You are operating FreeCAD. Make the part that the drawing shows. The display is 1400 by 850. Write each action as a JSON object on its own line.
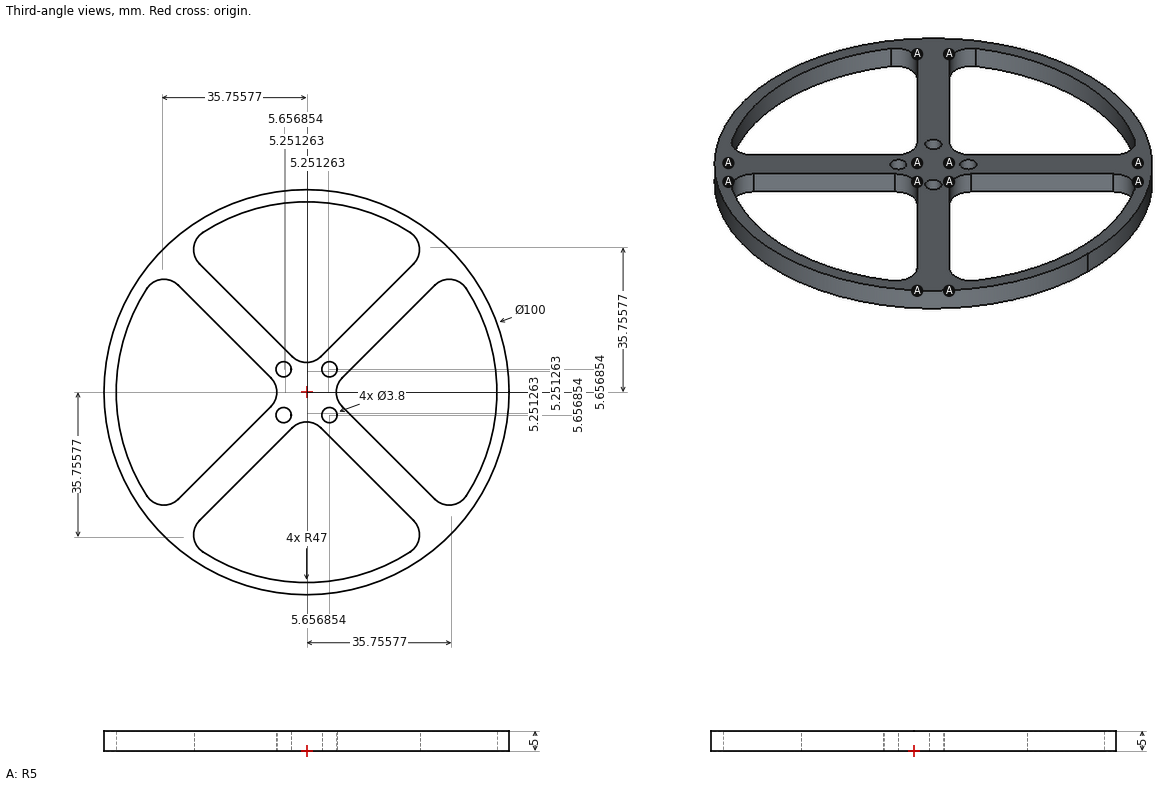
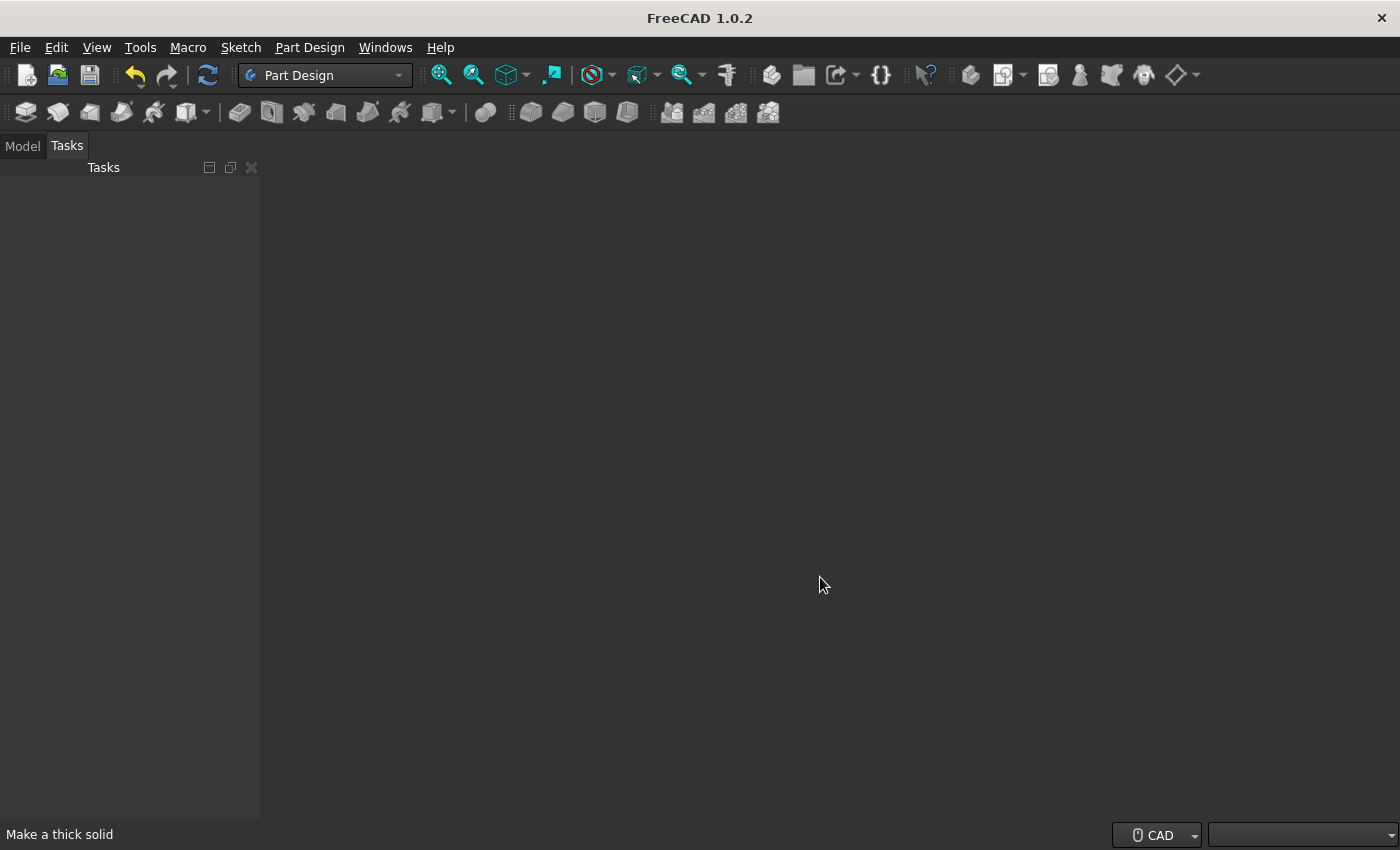
{"action": "left_click", "coordinate": [26, 76]}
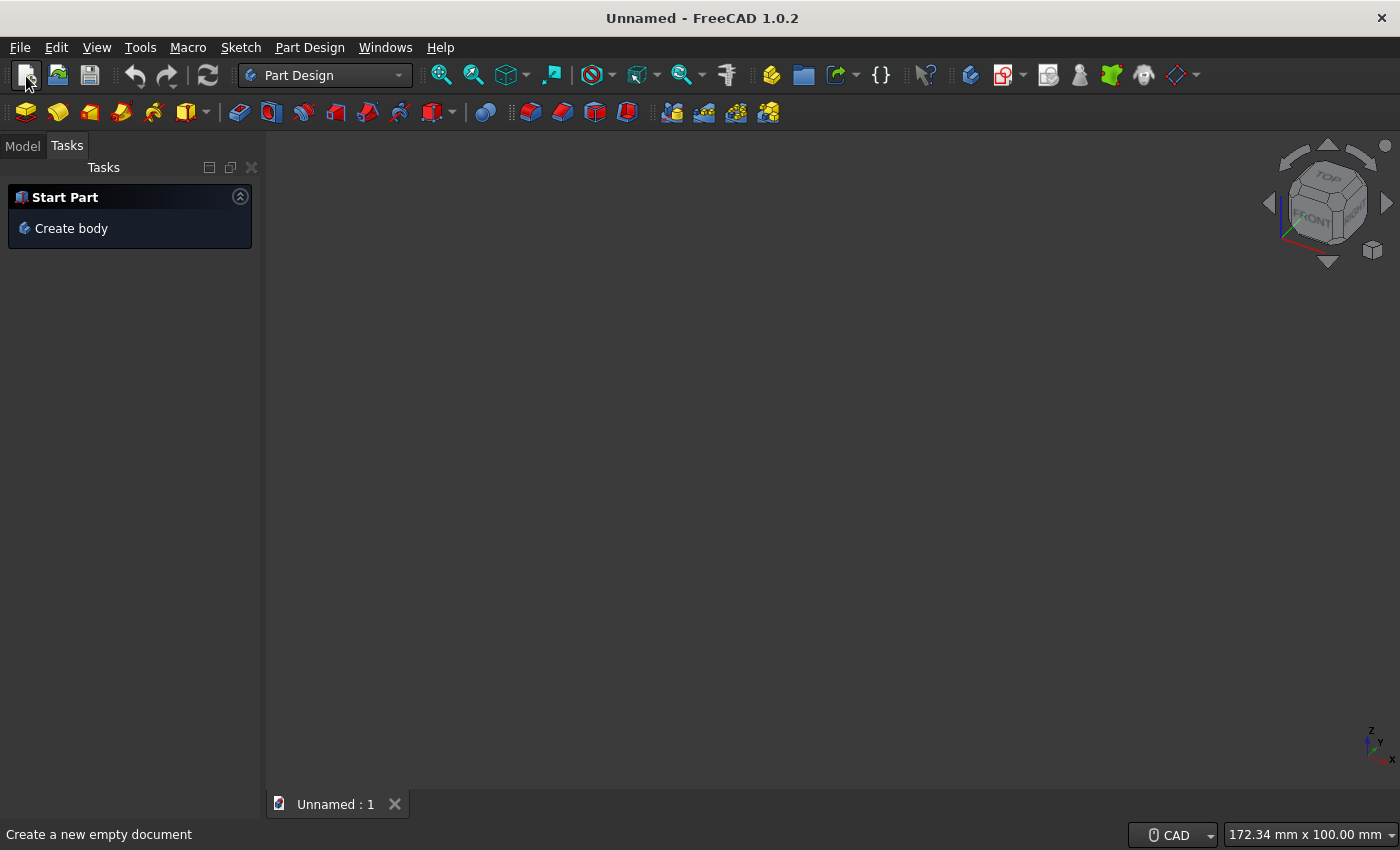
{"action": "left_click", "coordinate": [1004, 76]}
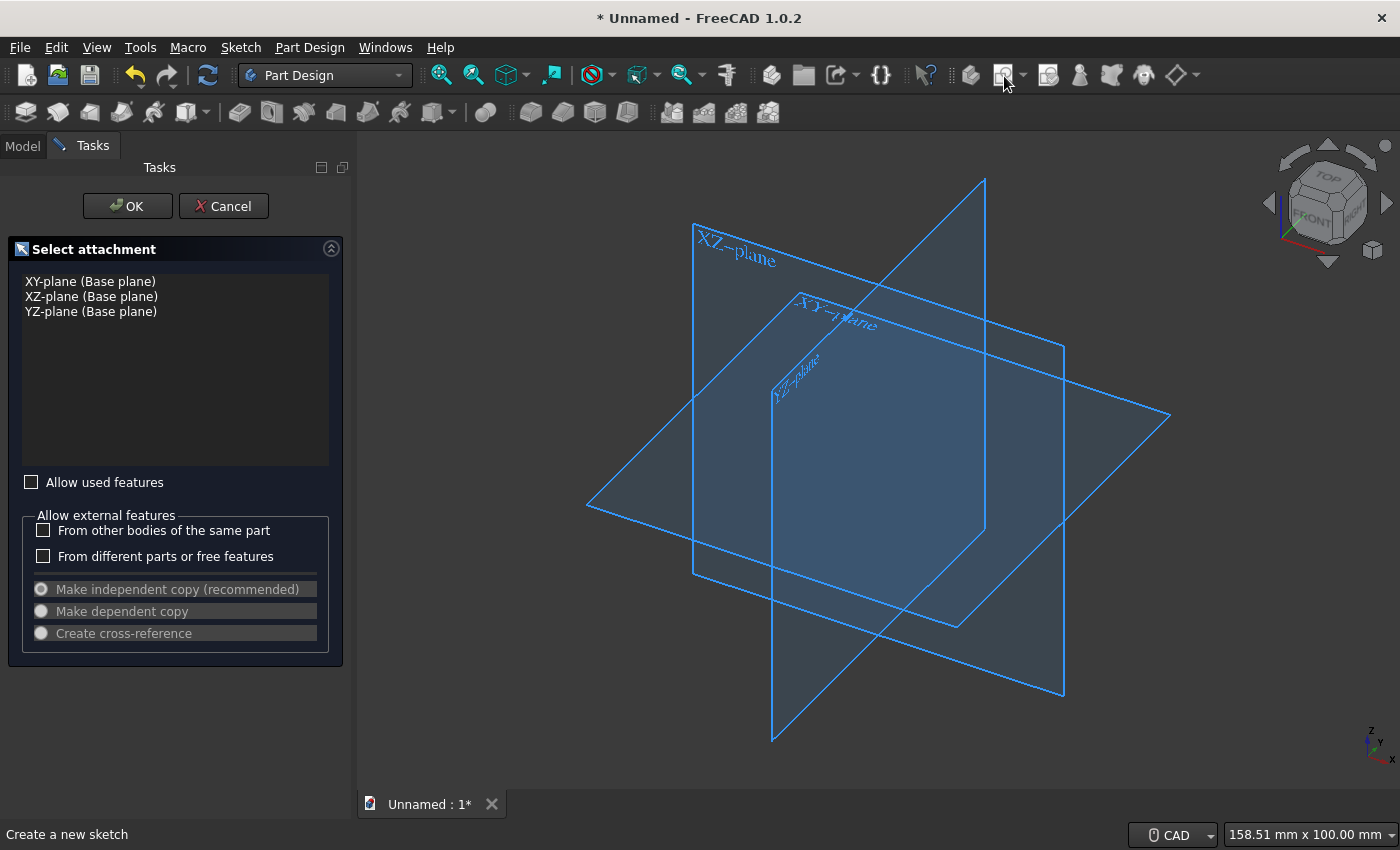
{"action": "left_click", "coordinate": [82, 282]}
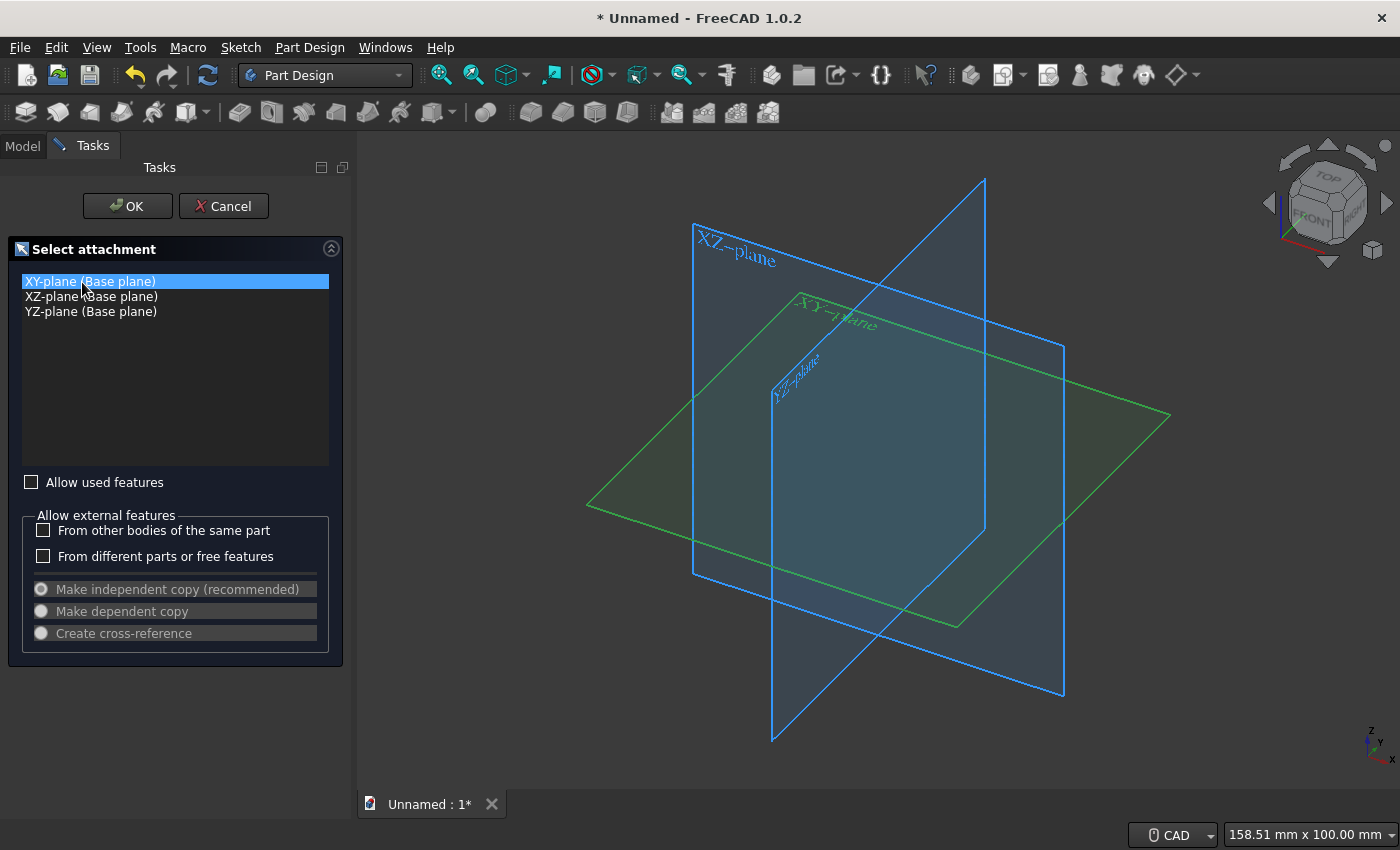
{"action": "left_click", "coordinate": [128, 206]}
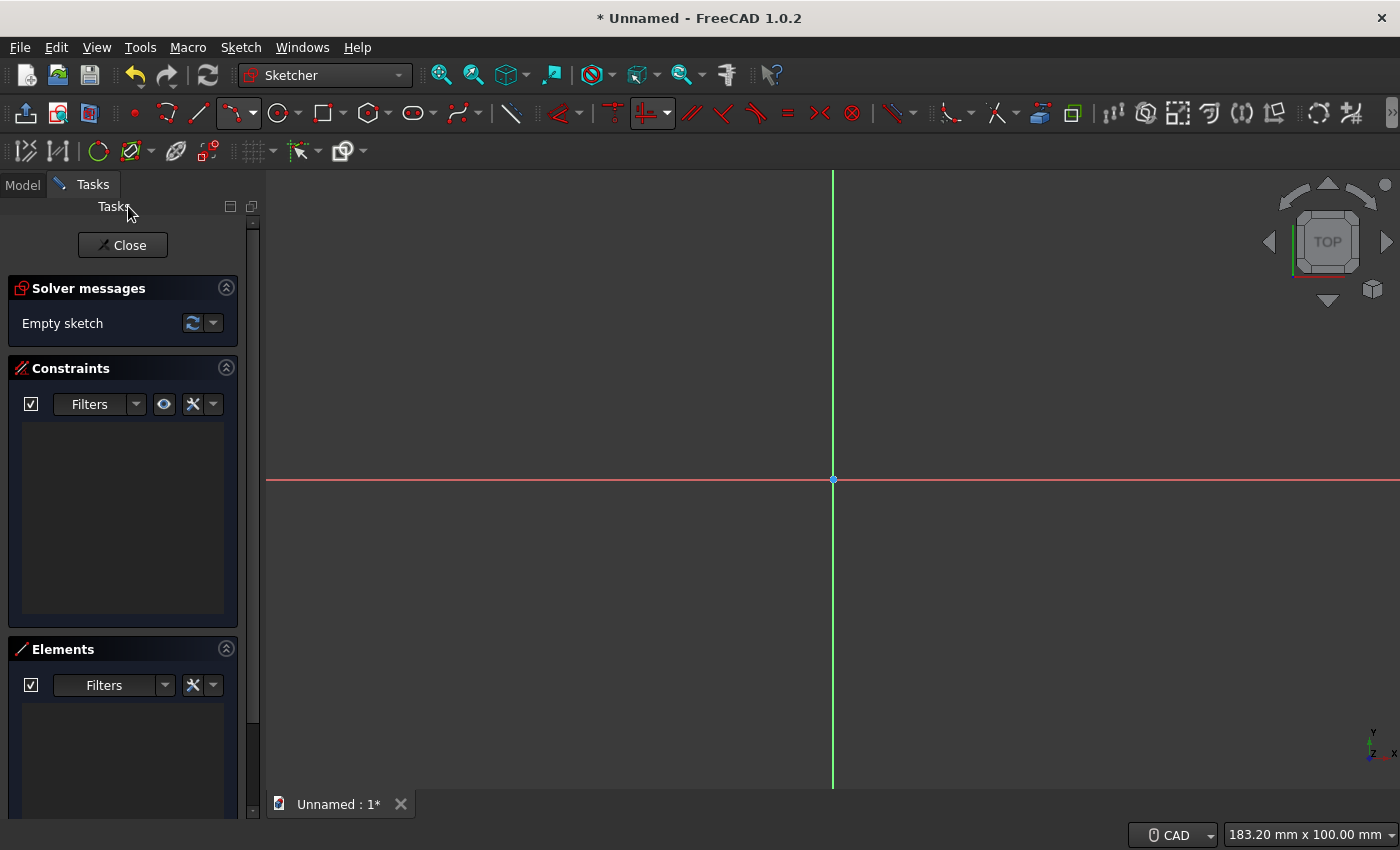
{"action": "scroll", "coordinate": [625, 480], "scroll_direction": "down", "scroll_amount": 2}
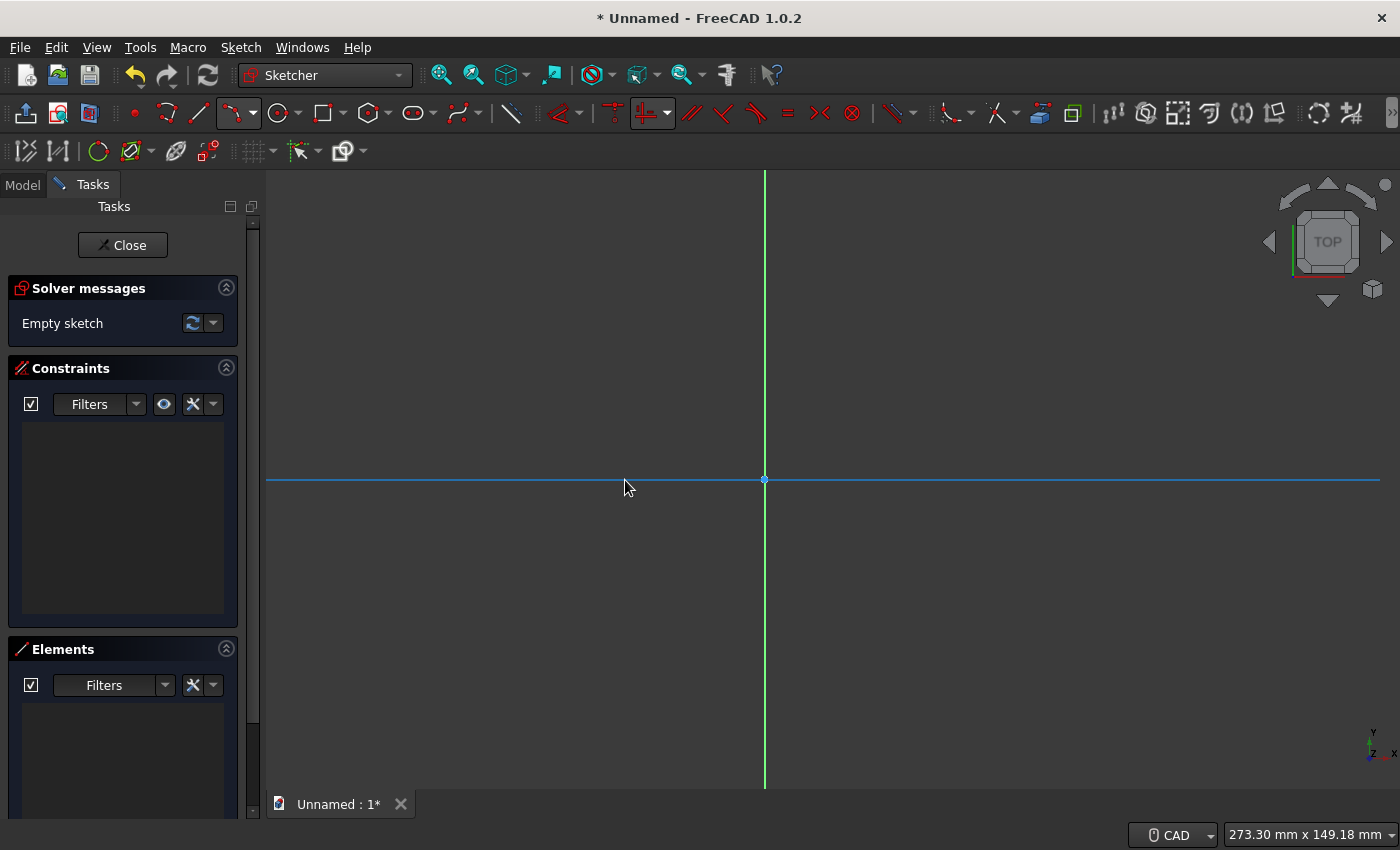
{"action": "left_click", "coordinate": [168, 114]}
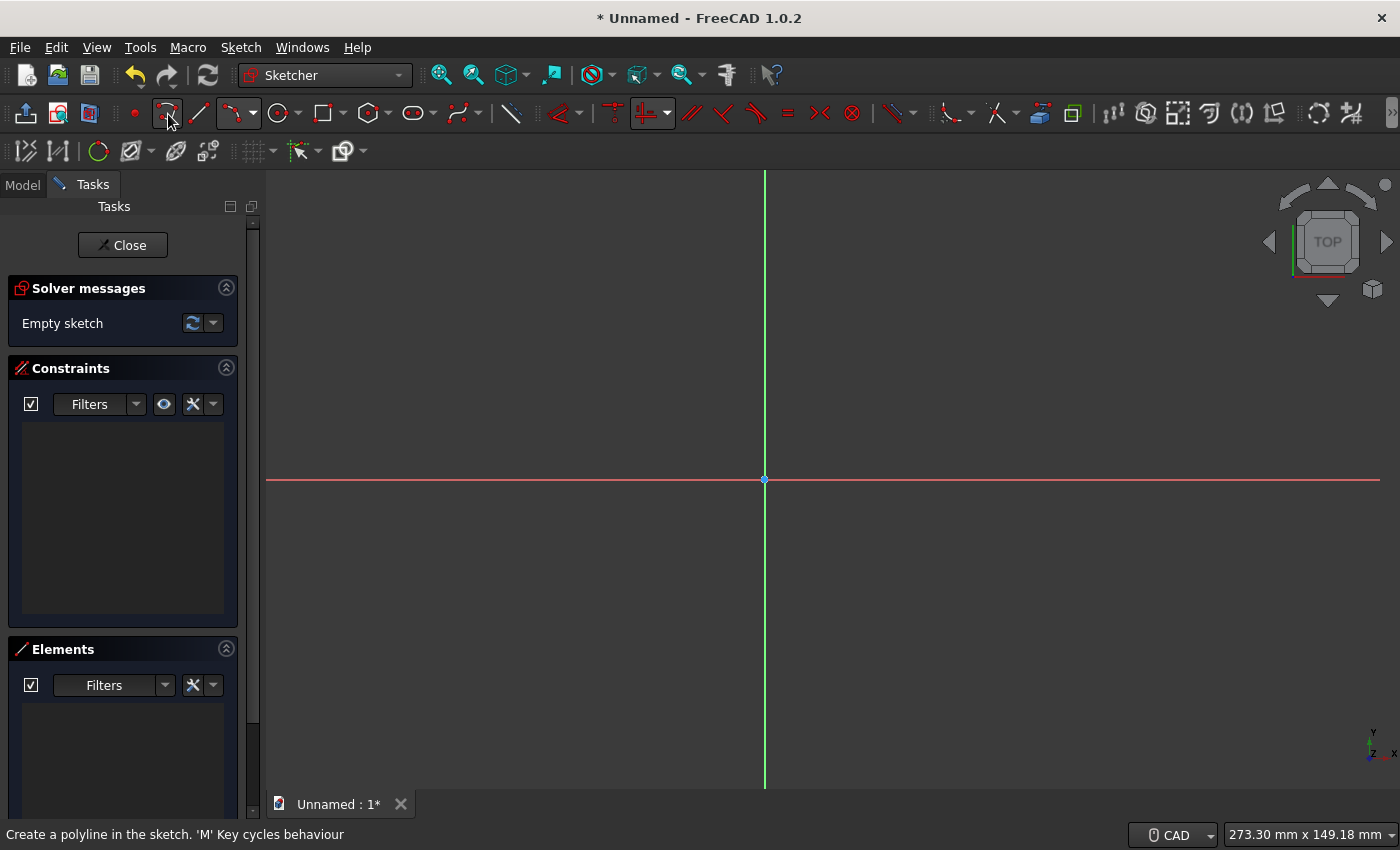
{"action": "left_click", "coordinate": [638, 628]}
{"action": "left_click", "coordinate": [765, 502]}
{"action": "left_click", "coordinate": [891, 628]}
{"action": "right_click", "coordinate": [891, 628]}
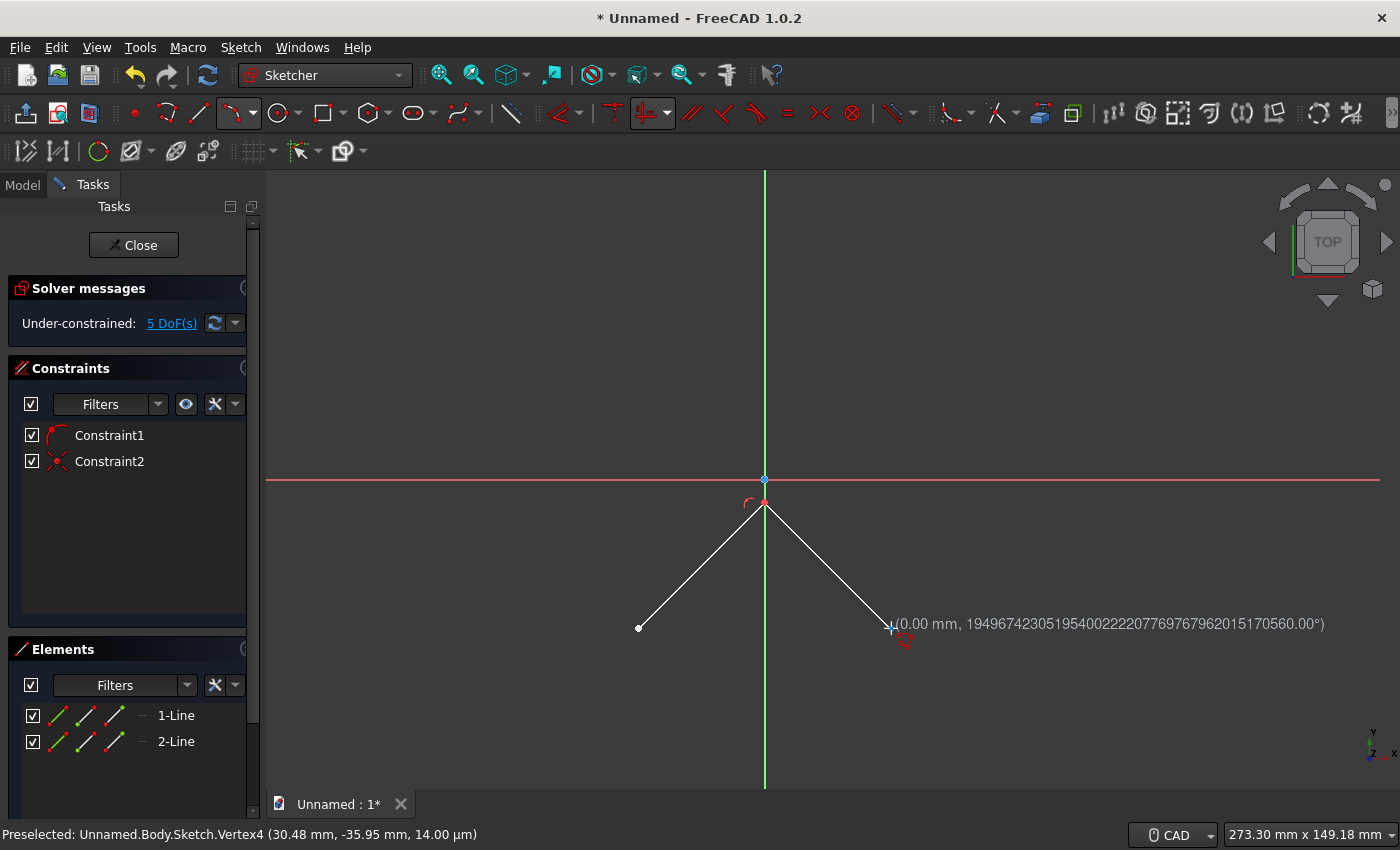
{"action": "left_click", "coordinate": [232, 114]}